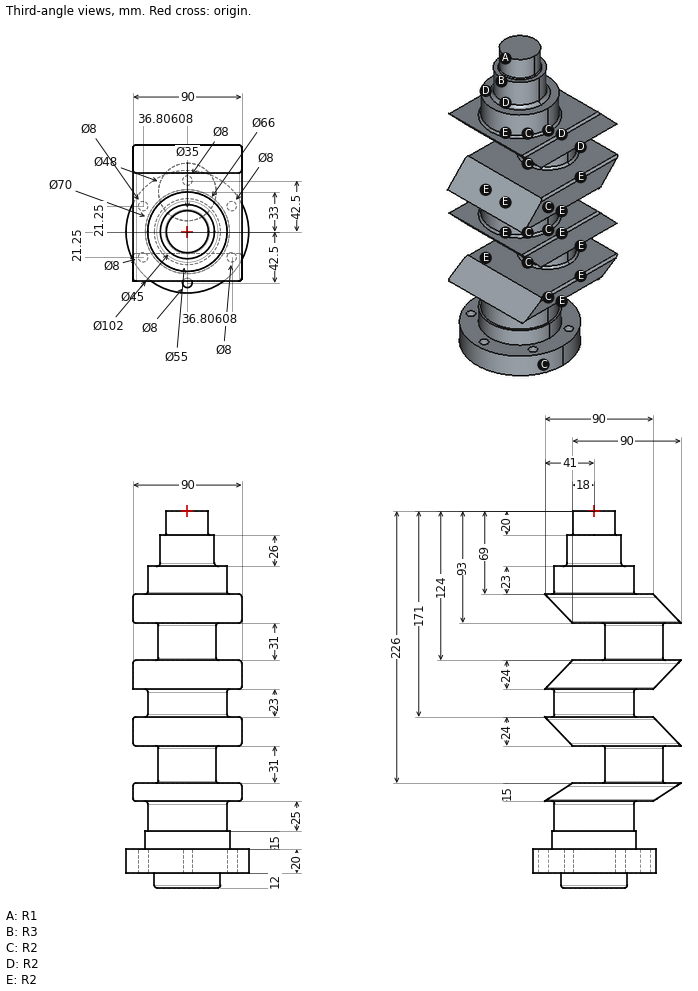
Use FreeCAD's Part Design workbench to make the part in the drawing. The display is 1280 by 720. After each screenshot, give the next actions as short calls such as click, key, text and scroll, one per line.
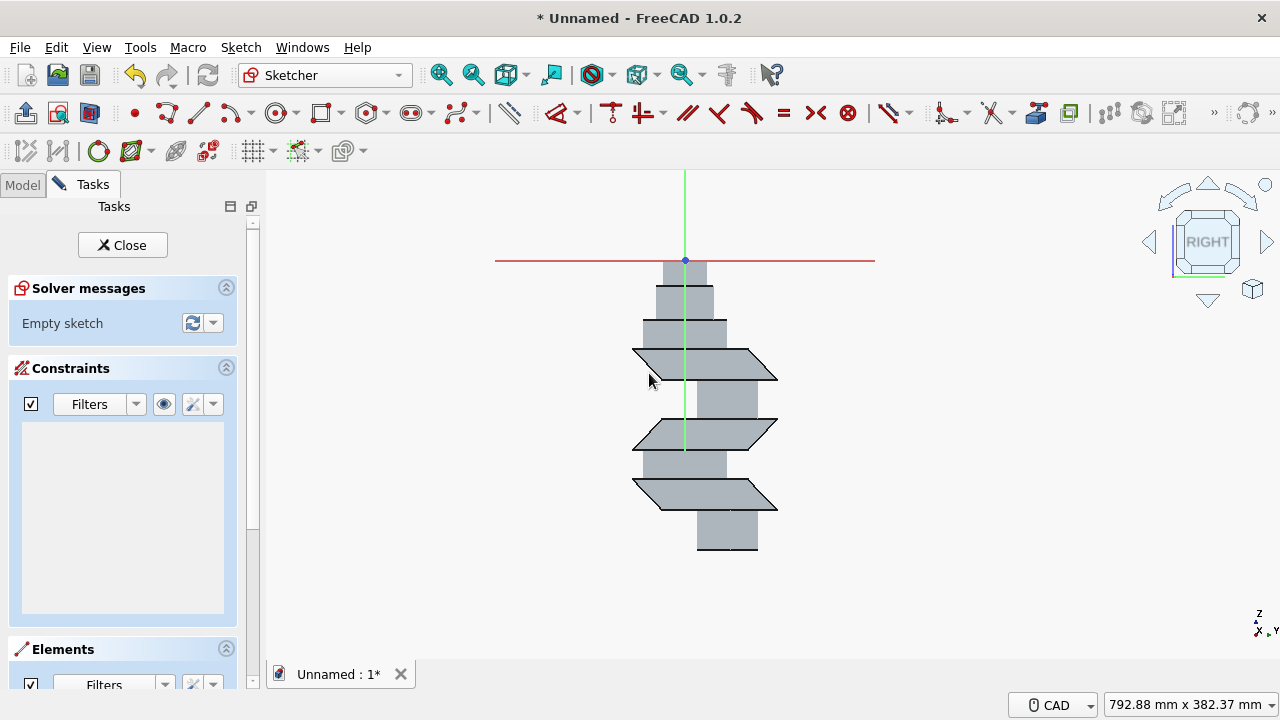
click(168, 114)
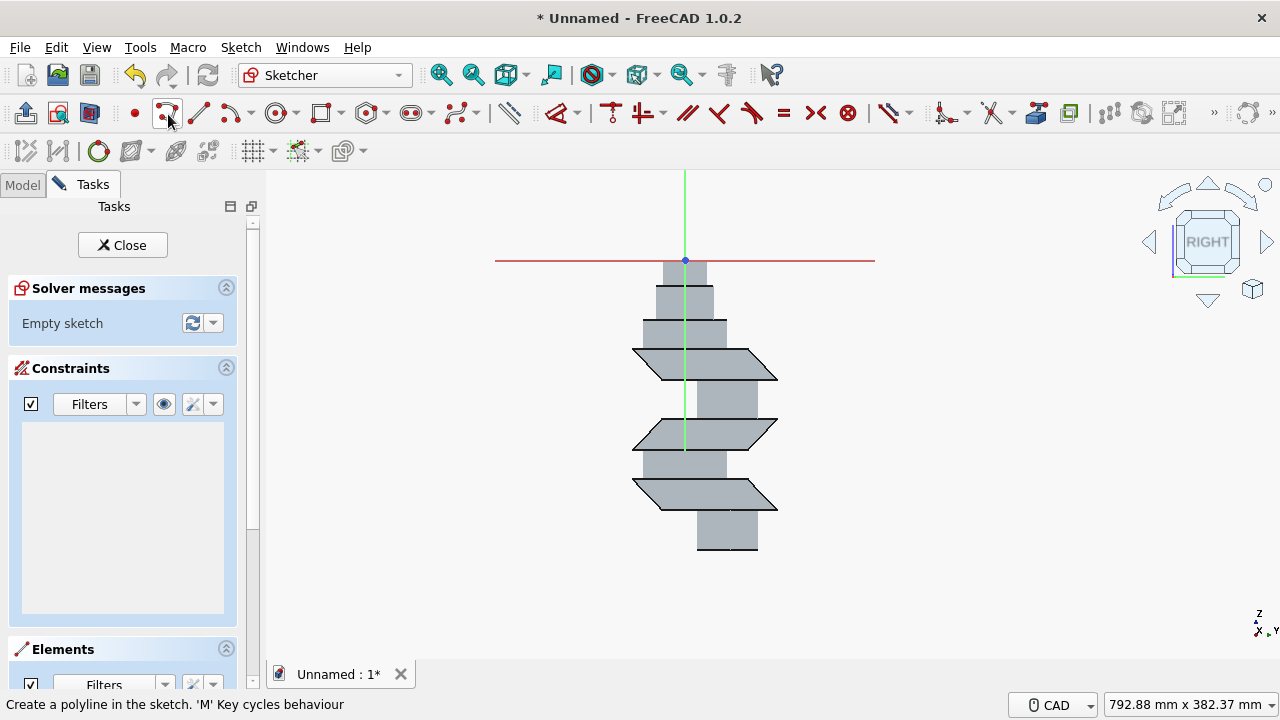
click(662, 550)
click(633, 569)
click(748, 569)
click(777, 550)
click(662, 551)
key(Escape)
key(Escape)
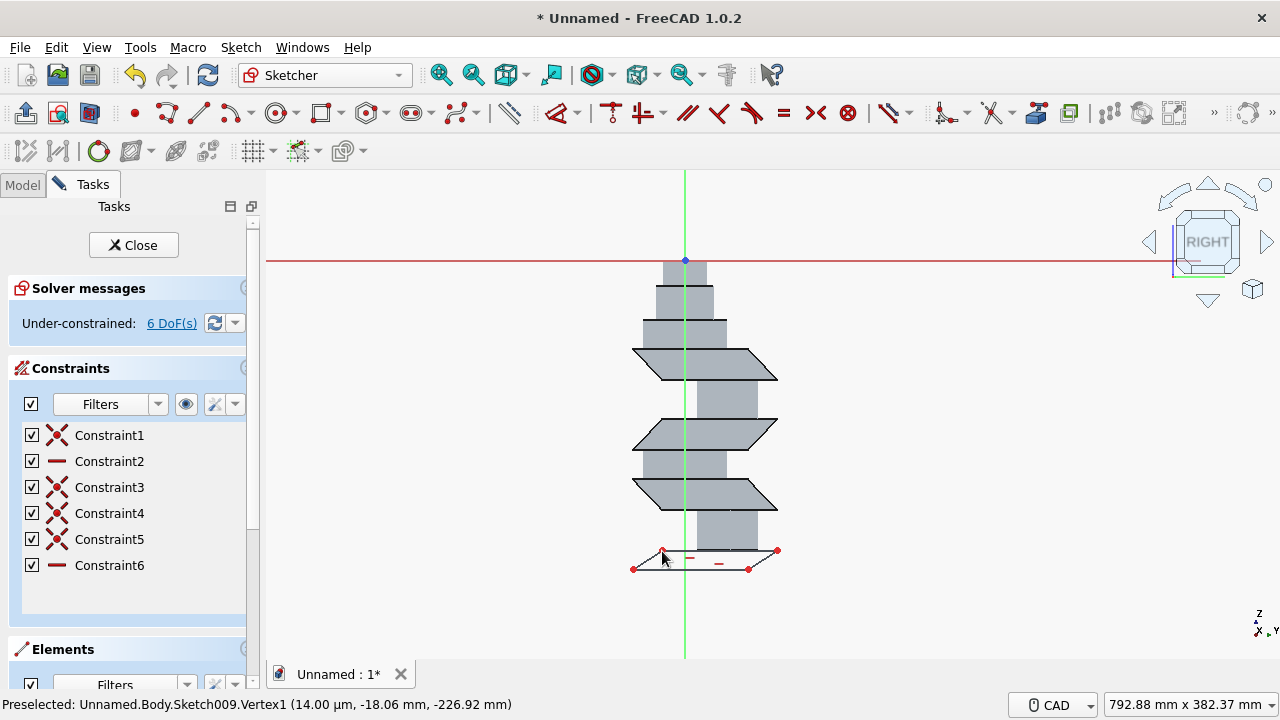
click(556, 114)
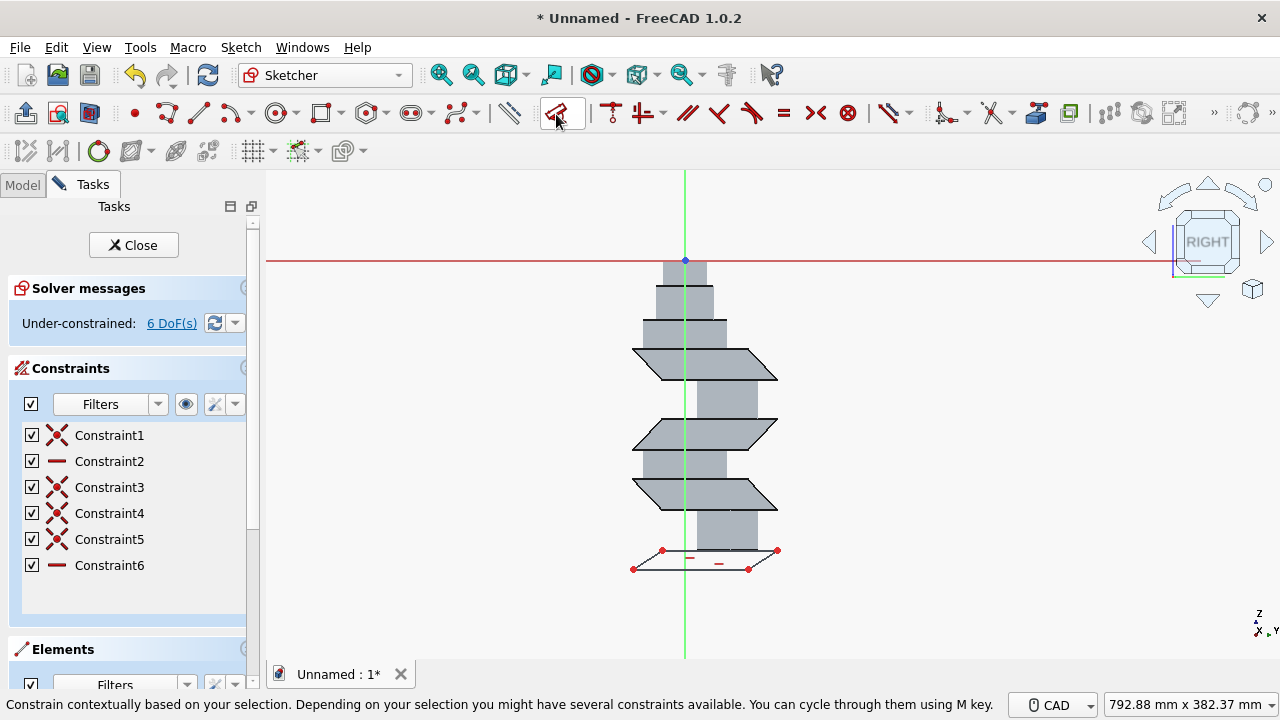
click(667, 570)
click(664, 604)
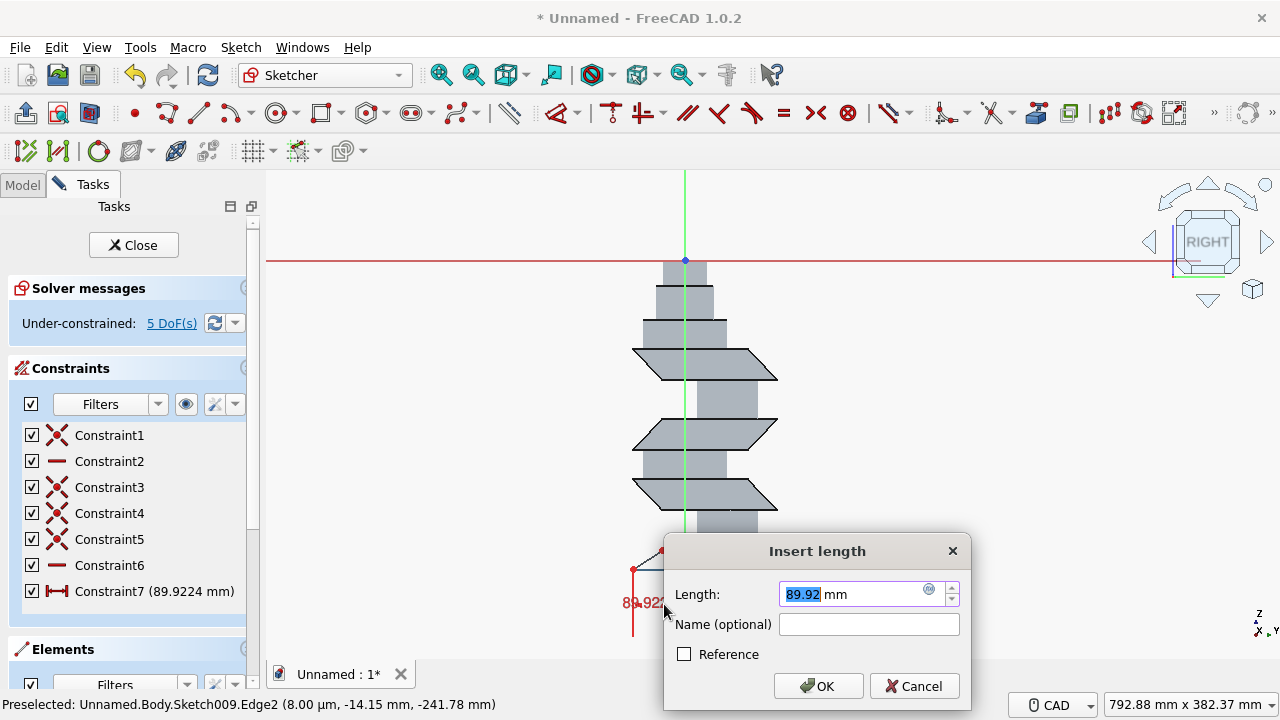
text(90)
key(Return)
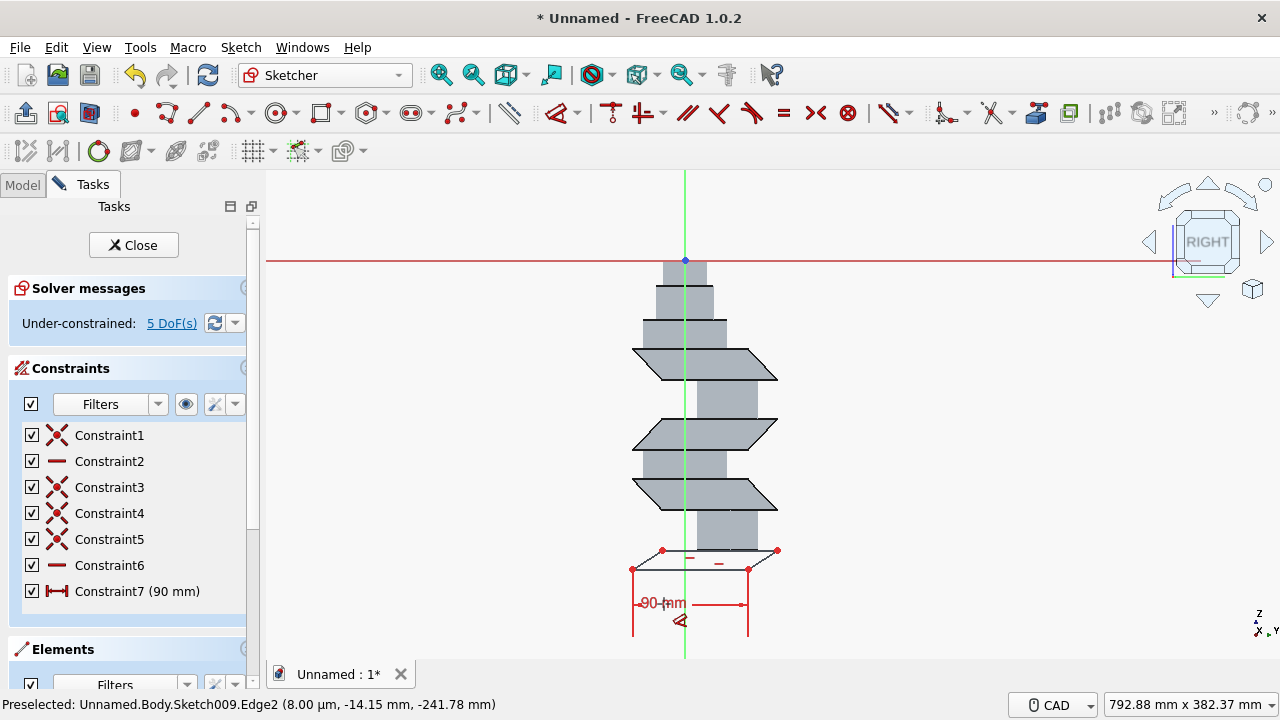
click(742, 551)
click(746, 585)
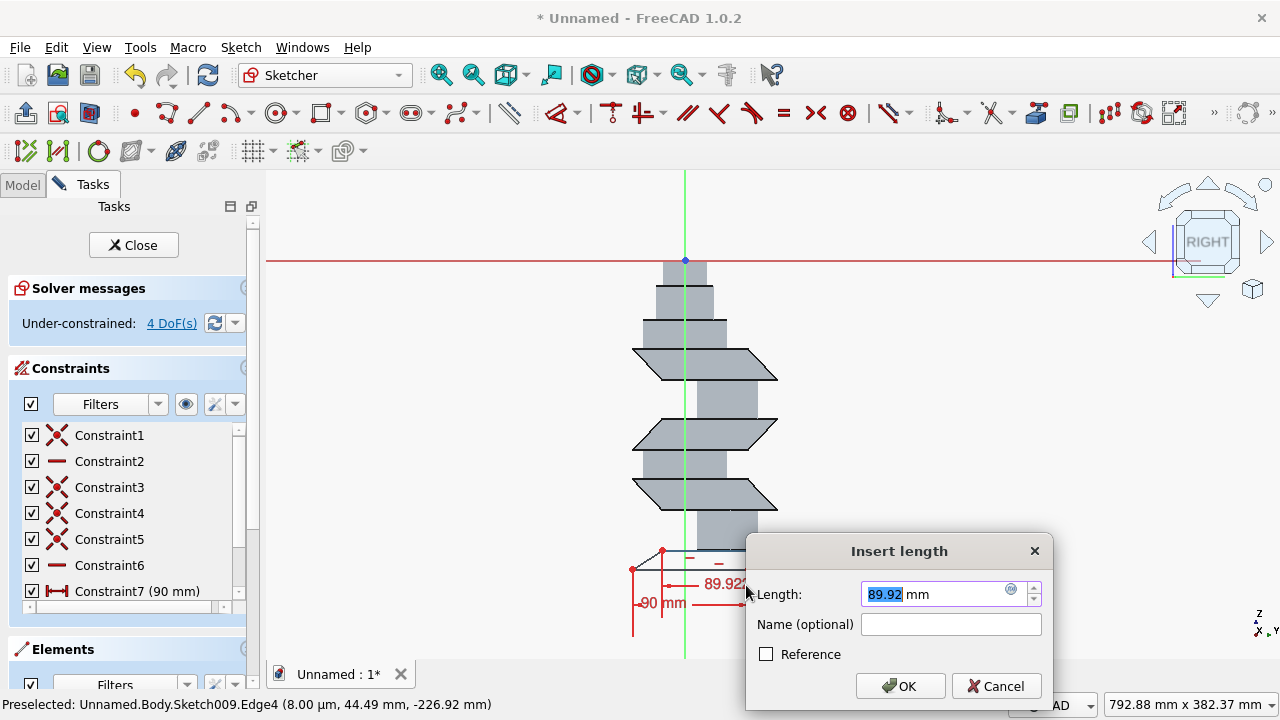
text(90)
key(Return)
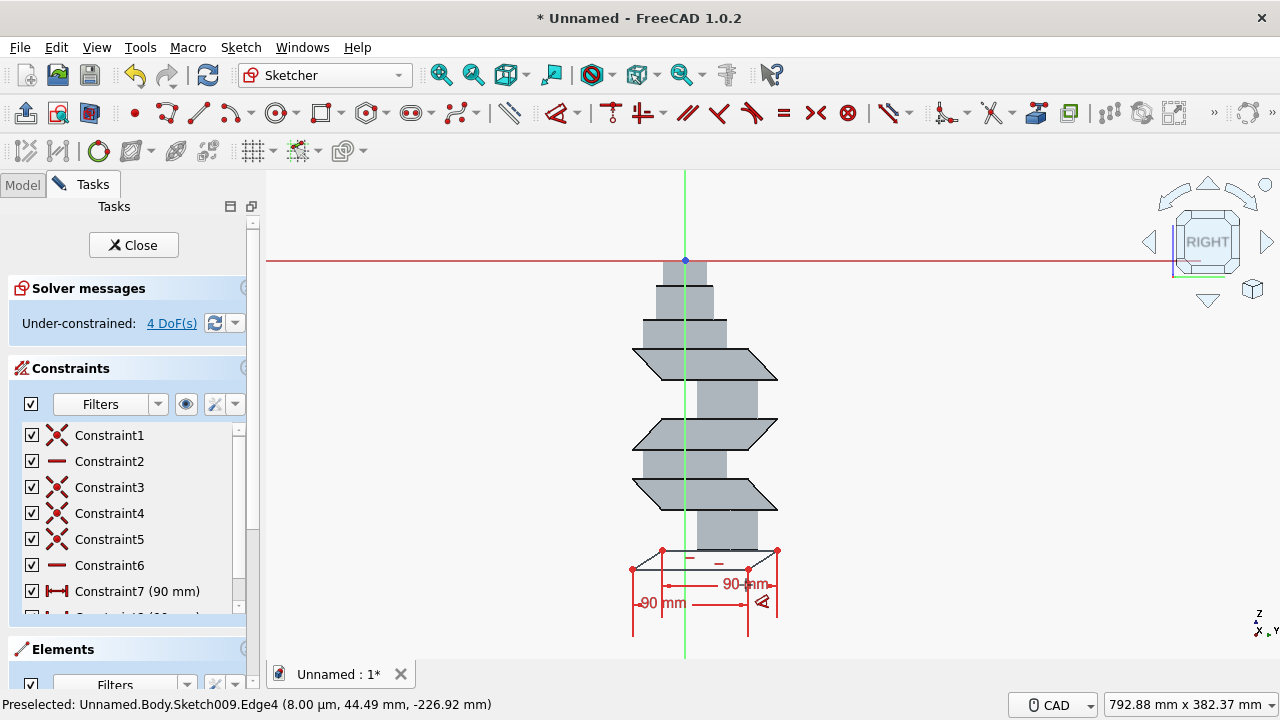
scroll(662, 551, up, 3)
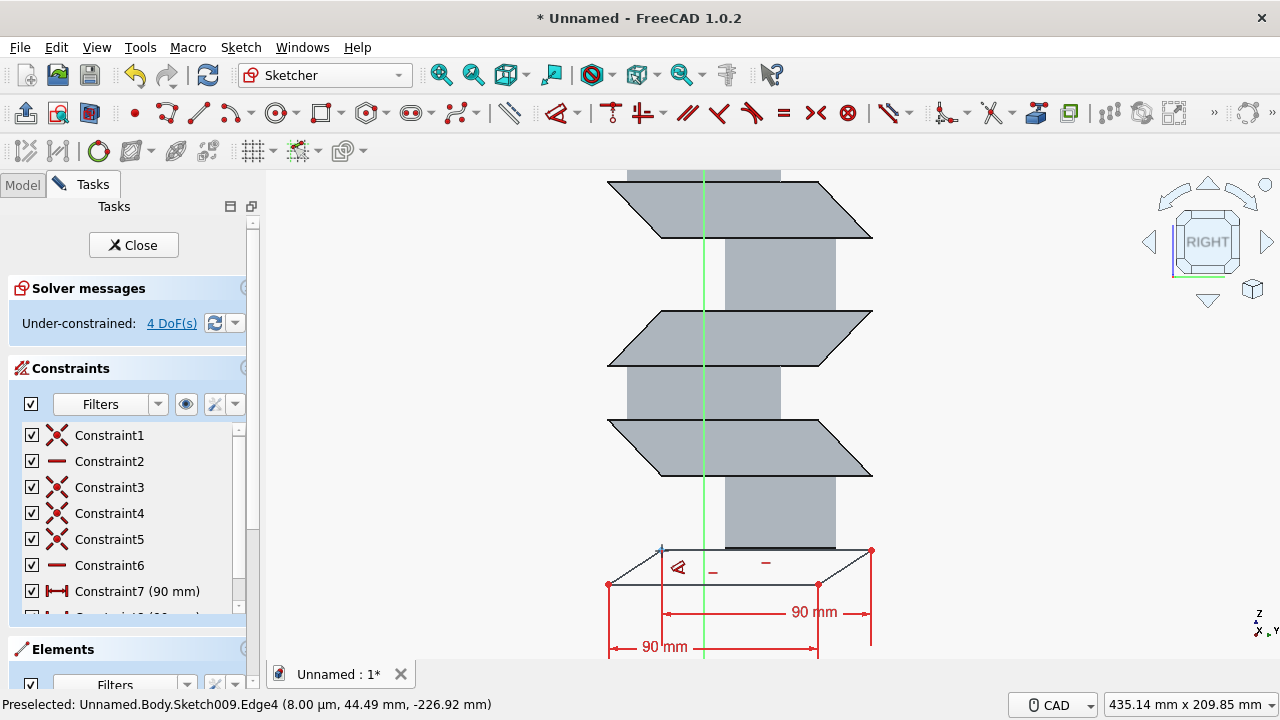
click(662, 550)
click(683, 608)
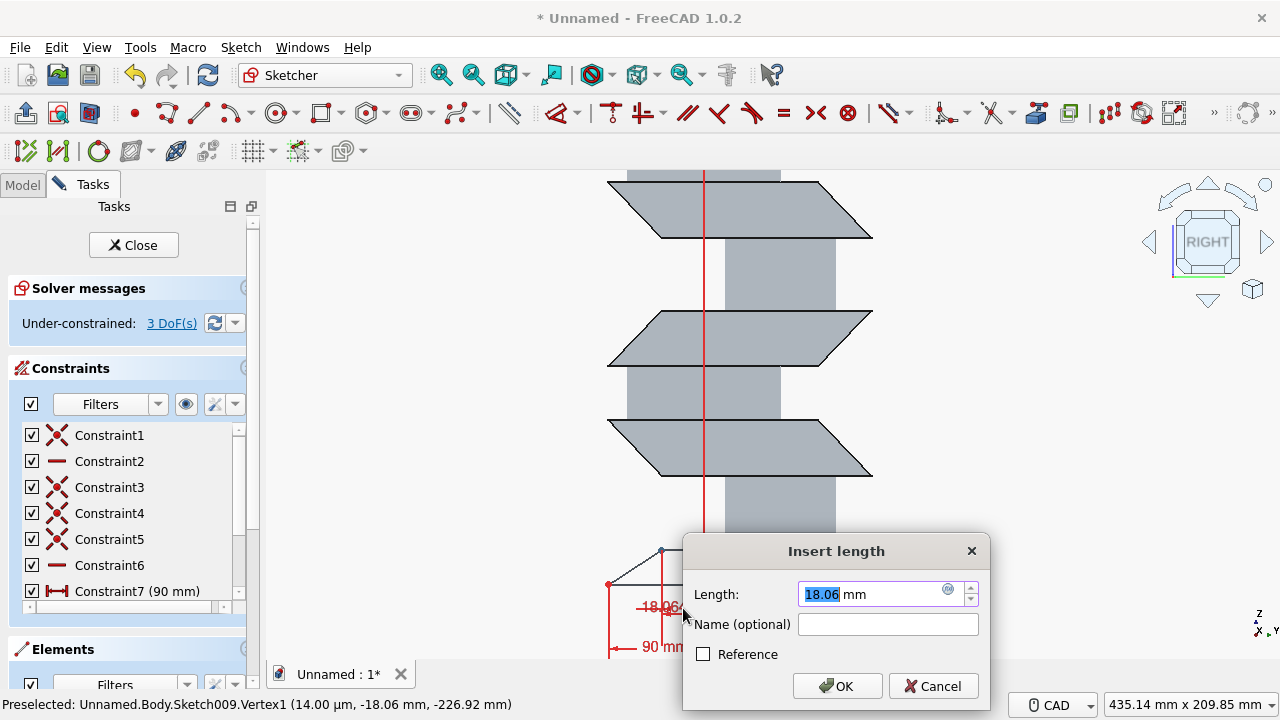
text(18)
key(Return)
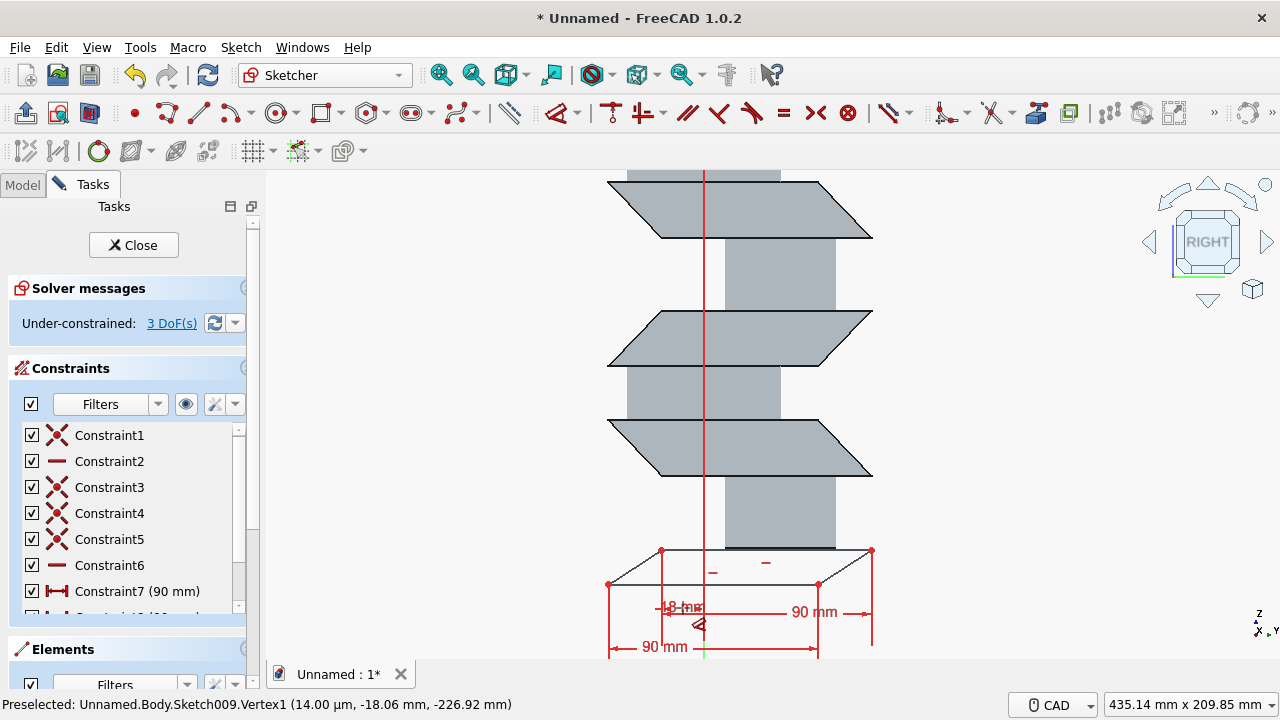
click(609, 585)
click(656, 619)